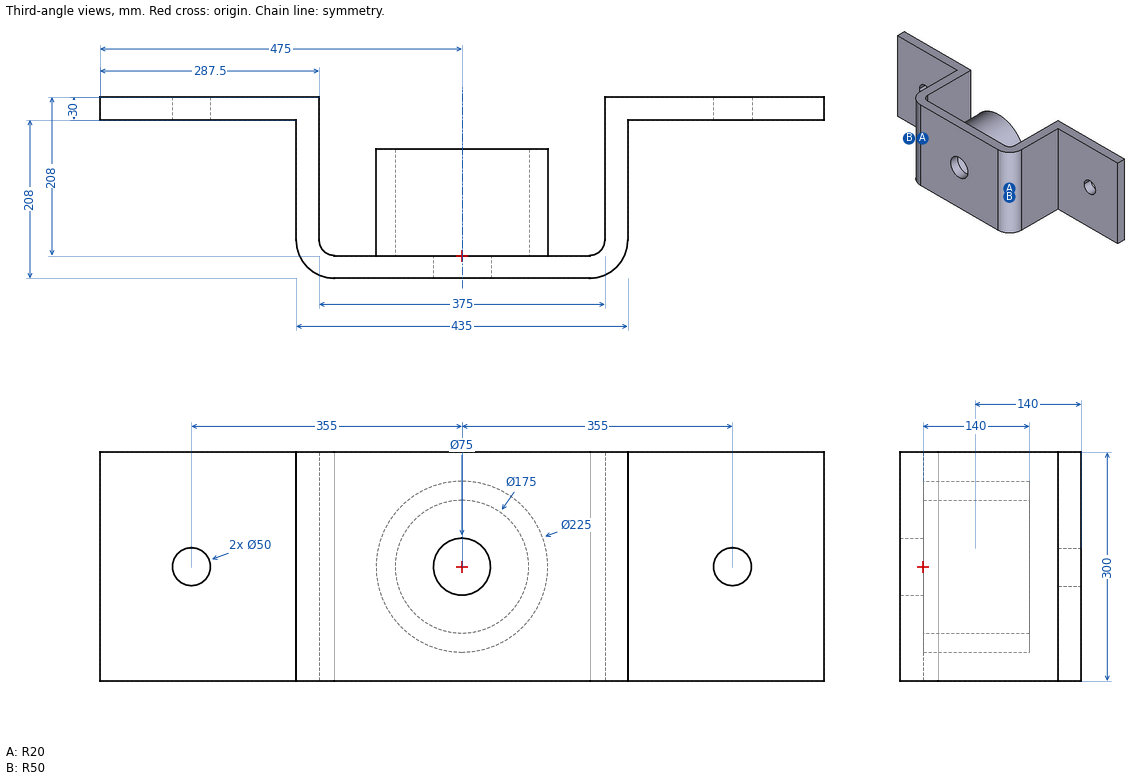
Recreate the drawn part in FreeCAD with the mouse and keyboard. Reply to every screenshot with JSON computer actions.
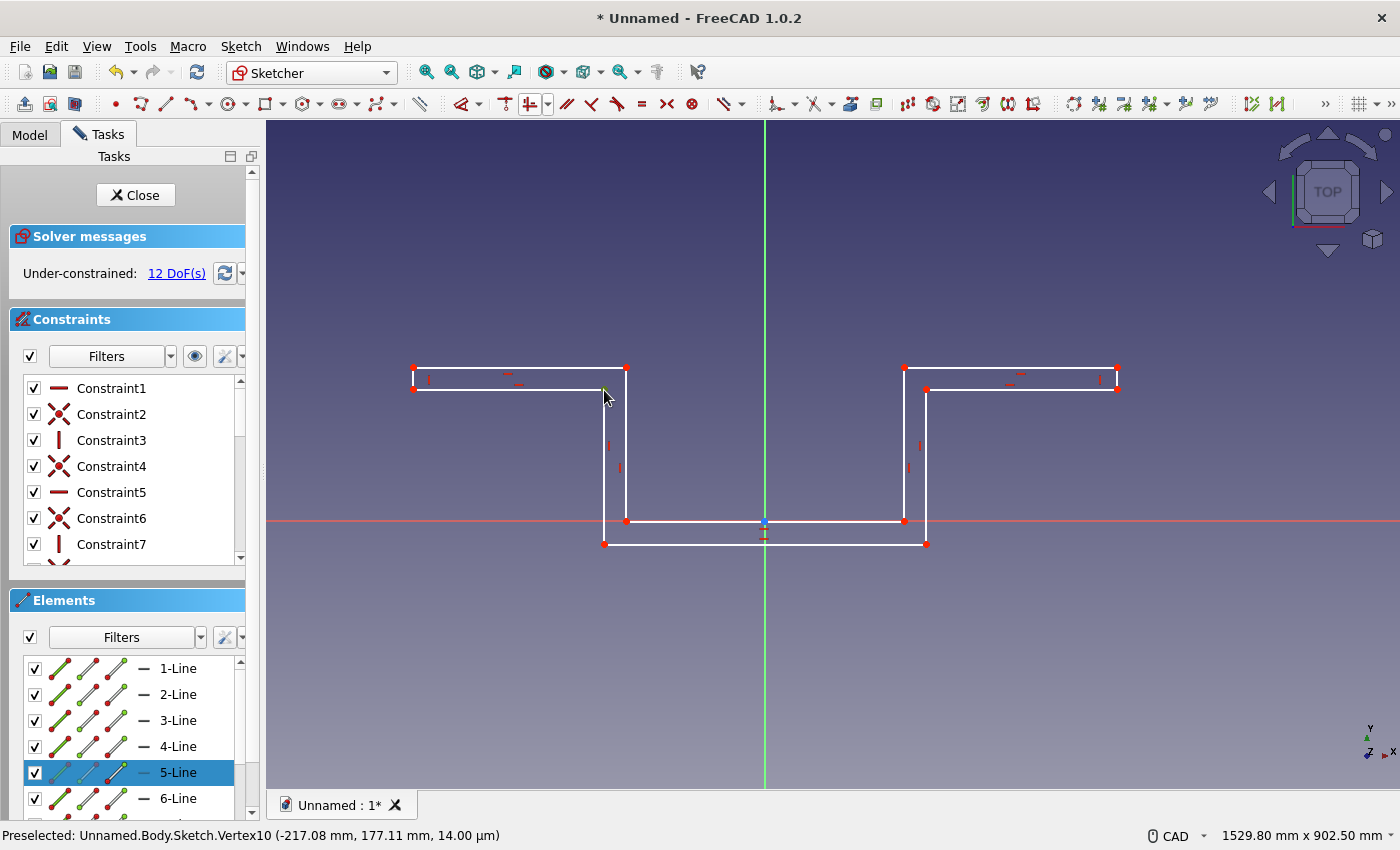
{"action": "left_click", "coordinate": [926, 390]}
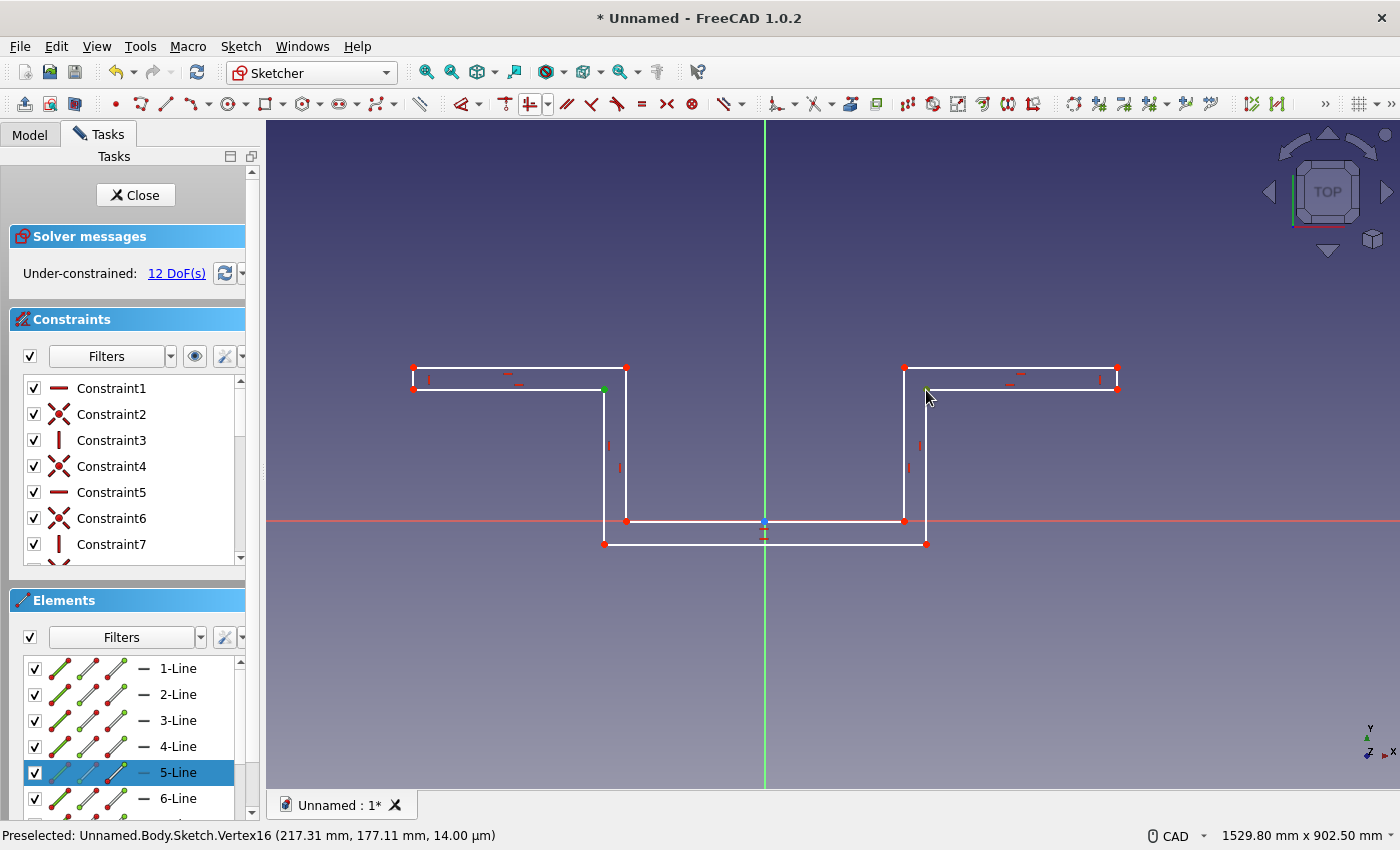
{"action": "left_click", "coordinate": [765, 717]}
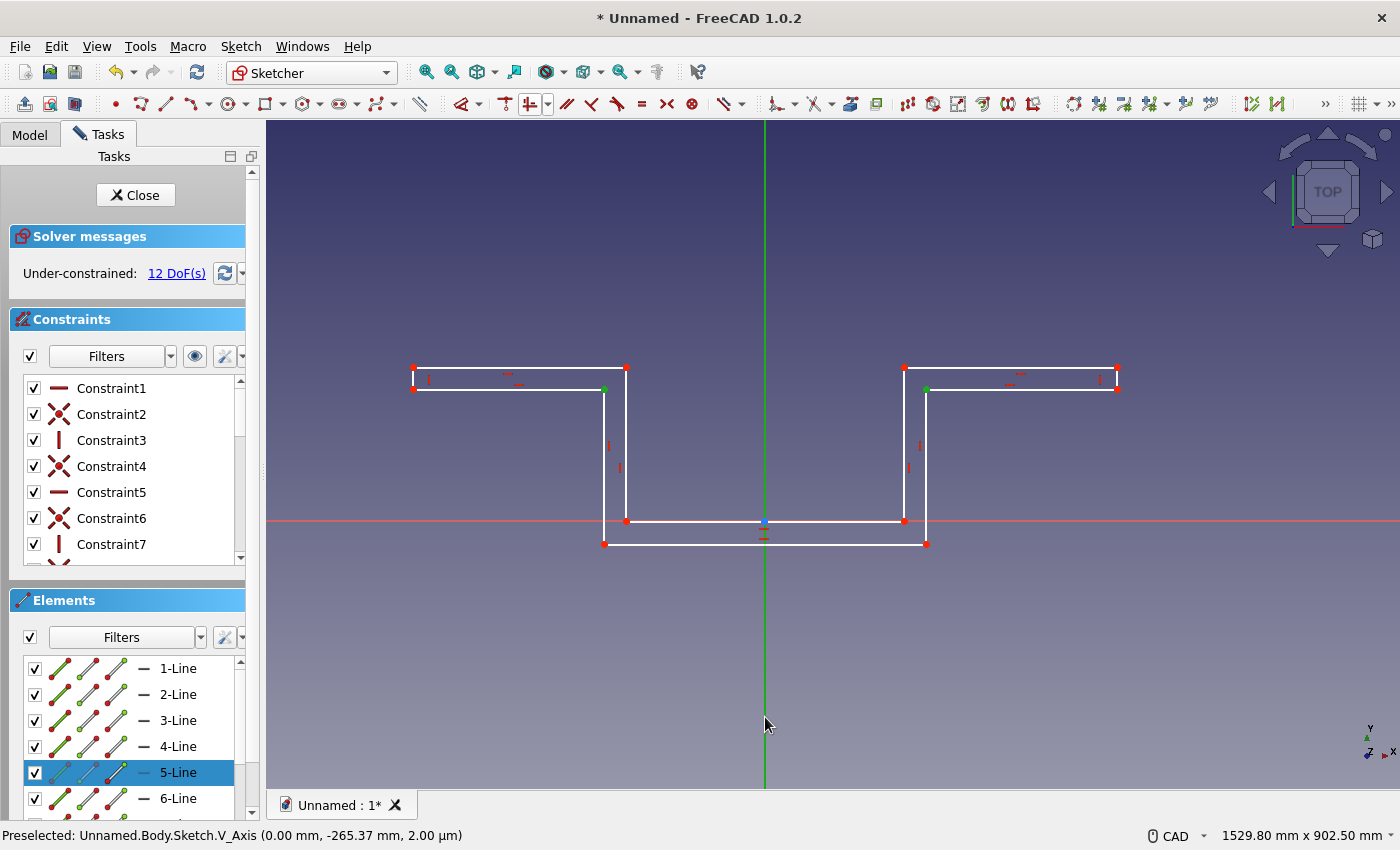
{"action": "left_click", "coordinate": [667, 104]}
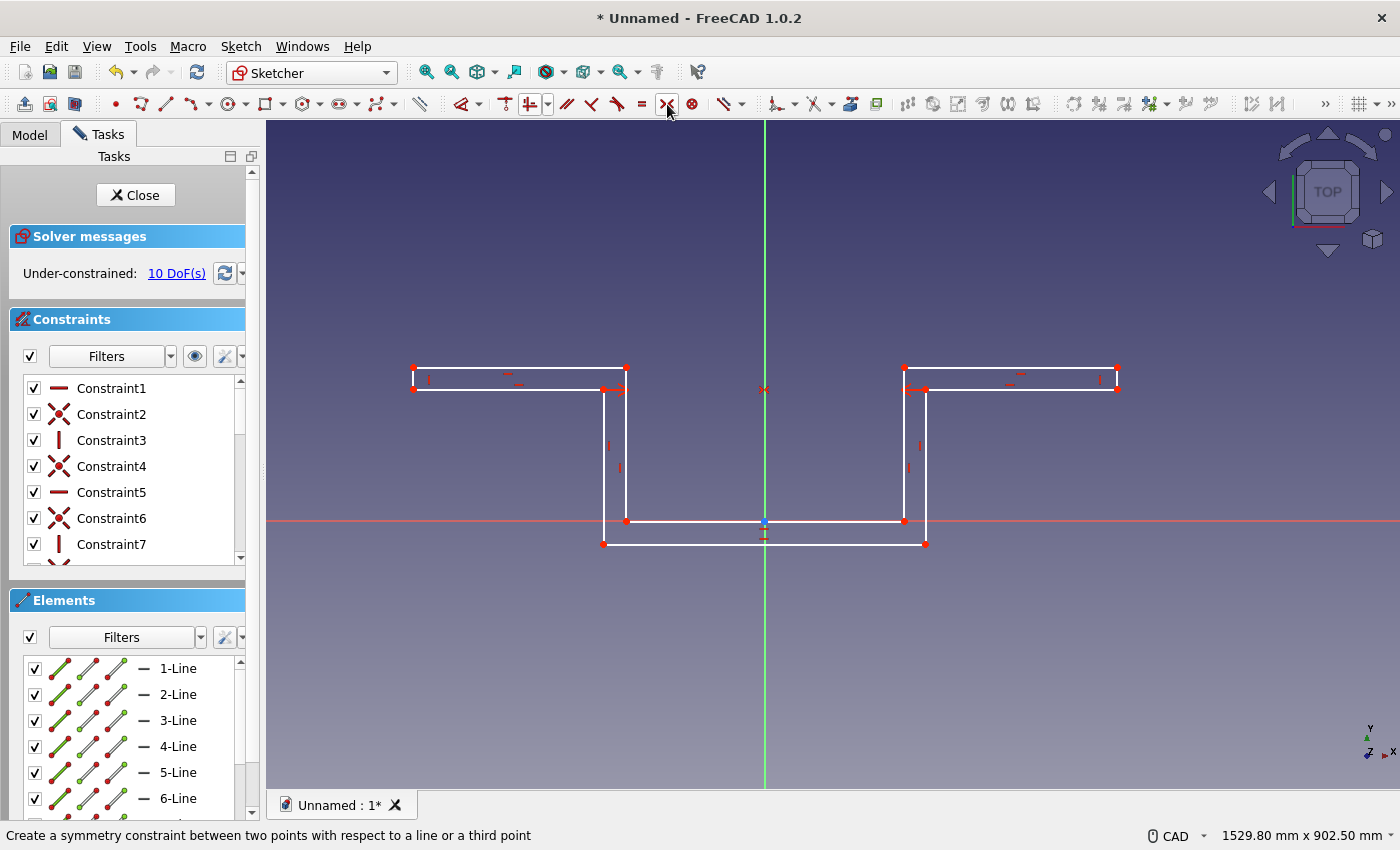
{"action": "left_click", "coordinate": [413, 368]}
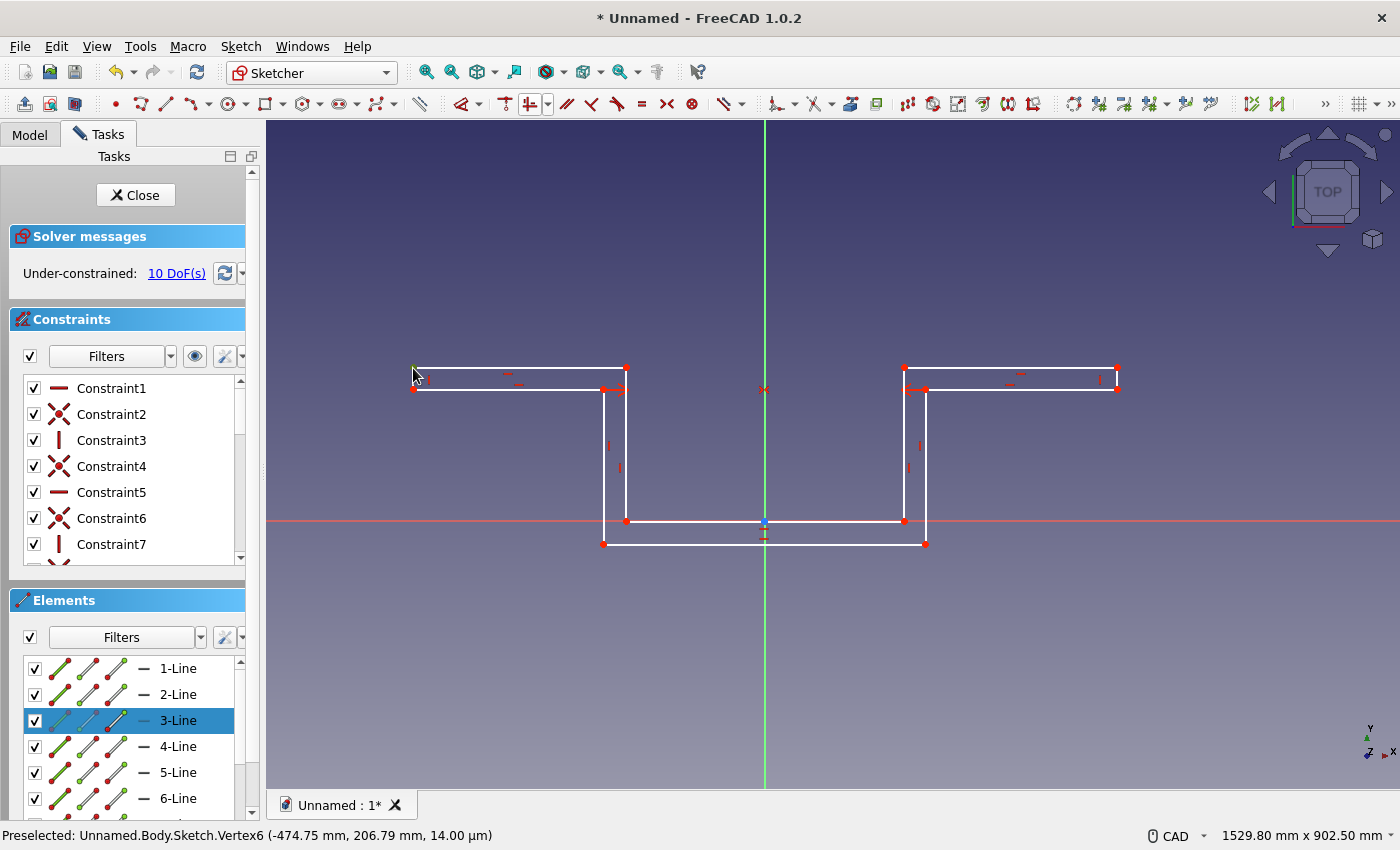
{"action": "left_click", "coordinate": [1117, 368]}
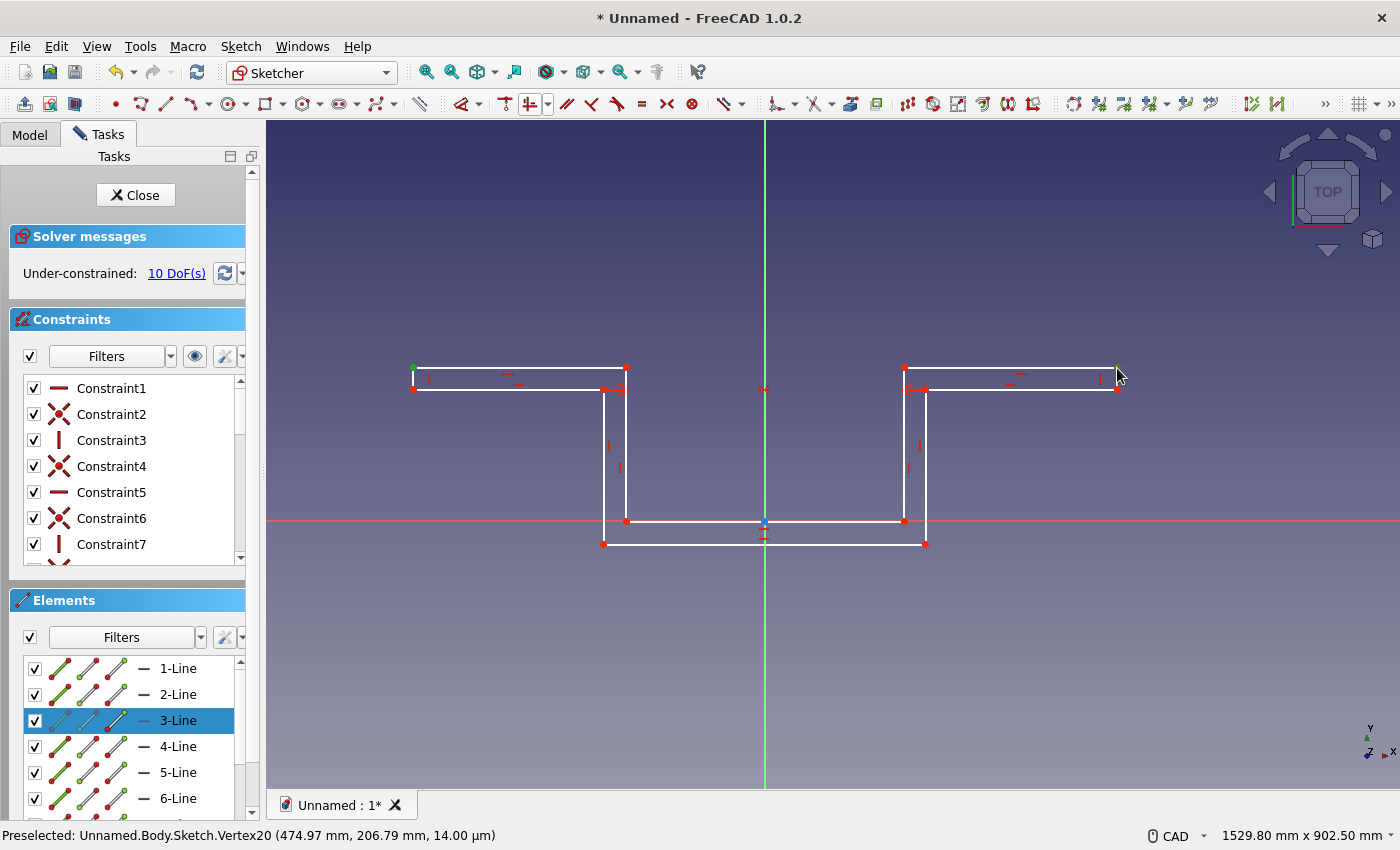
{"action": "left_click", "coordinate": [765, 717]}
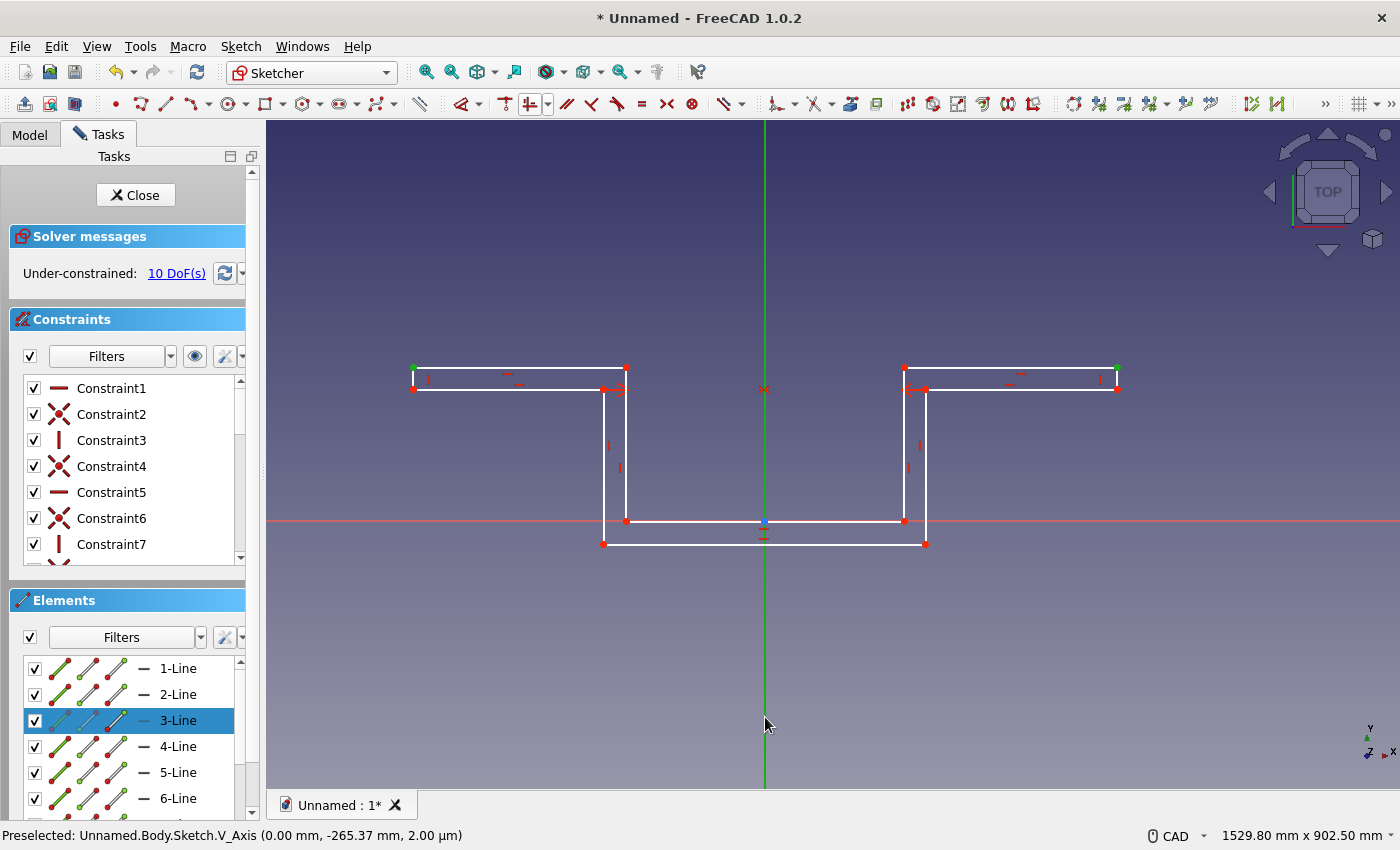
{"action": "left_click", "coordinate": [667, 104]}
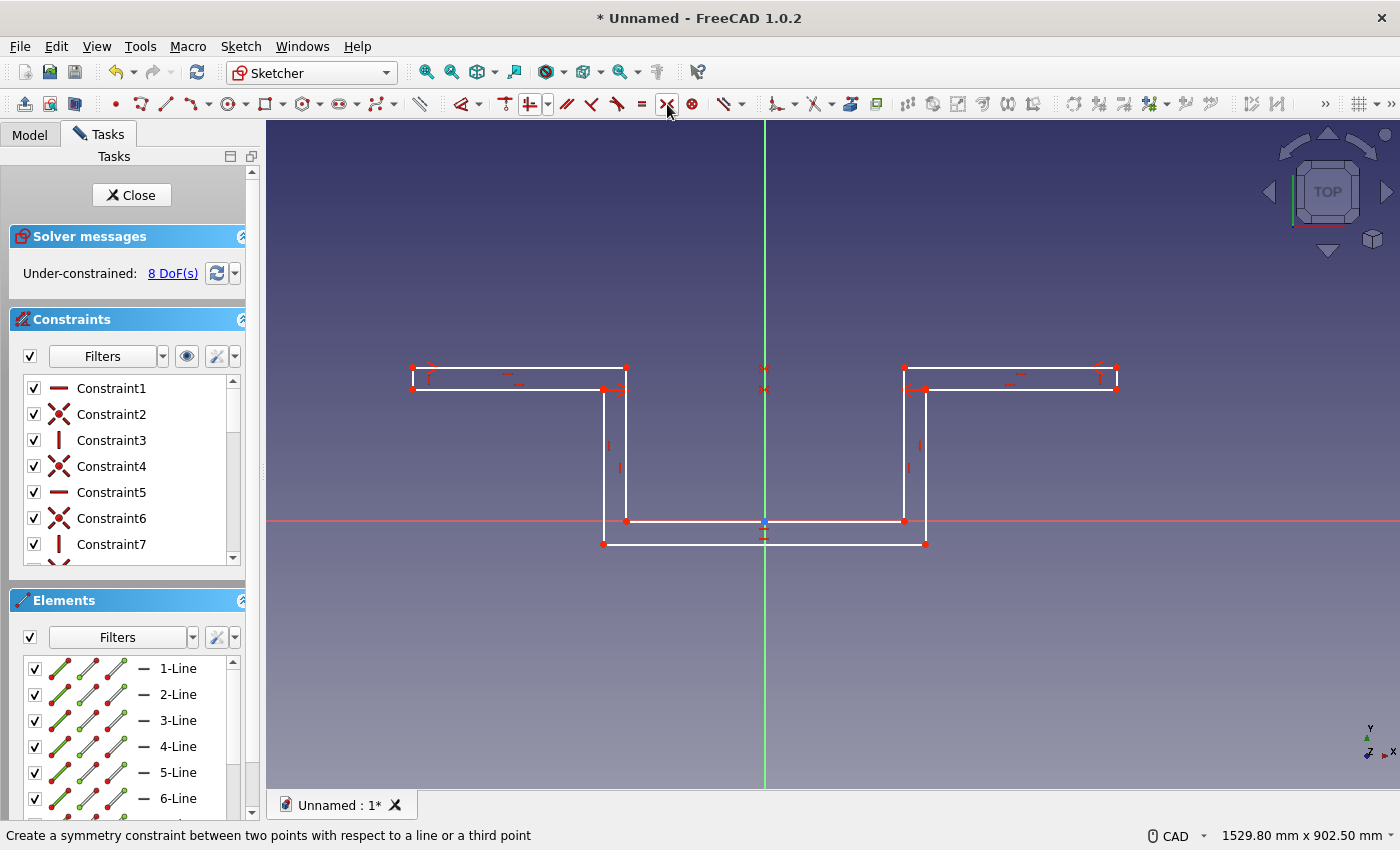
{"action": "left_click", "coordinate": [904, 522]}